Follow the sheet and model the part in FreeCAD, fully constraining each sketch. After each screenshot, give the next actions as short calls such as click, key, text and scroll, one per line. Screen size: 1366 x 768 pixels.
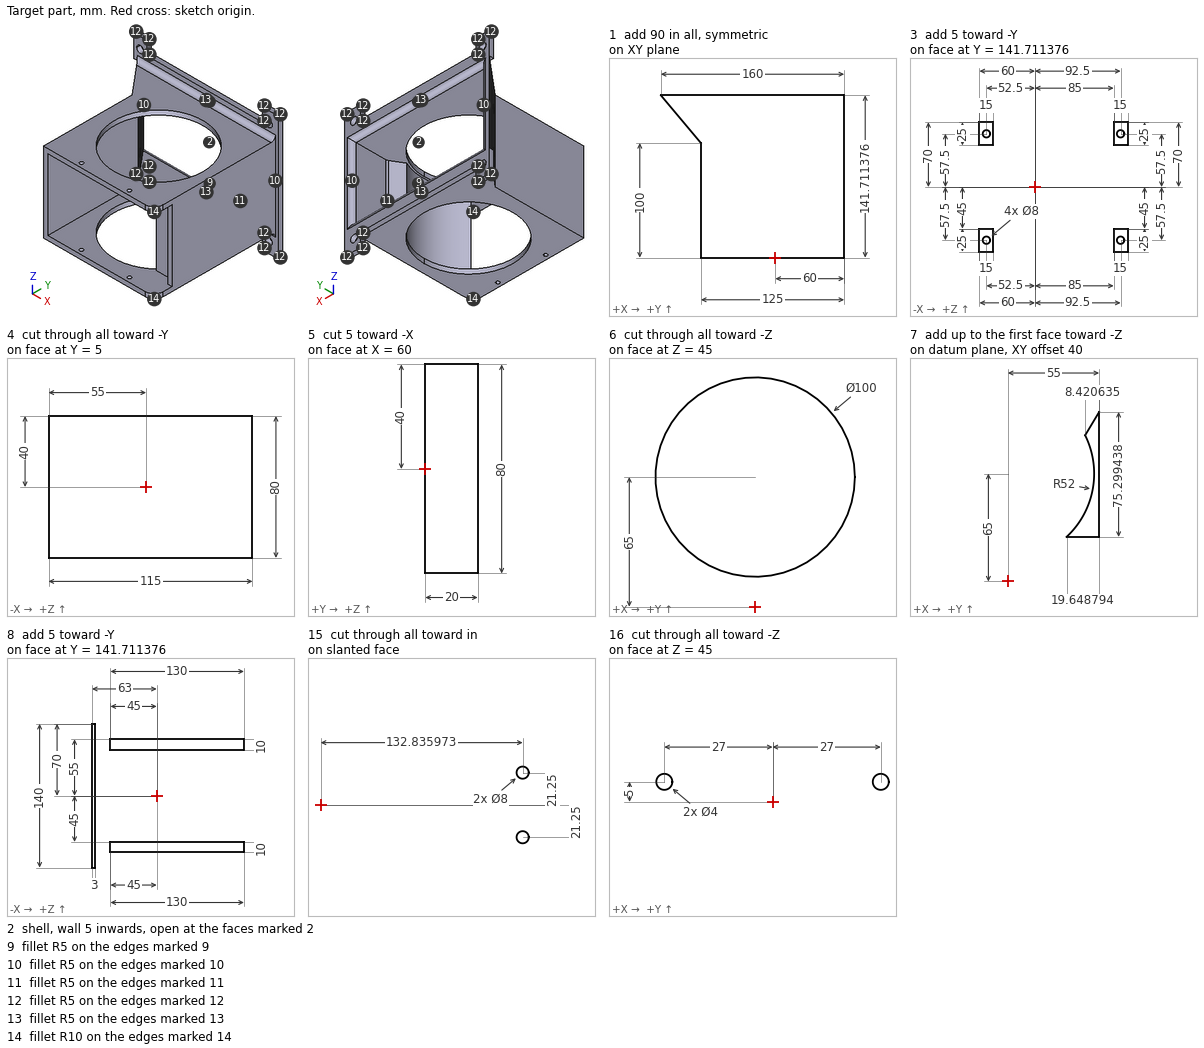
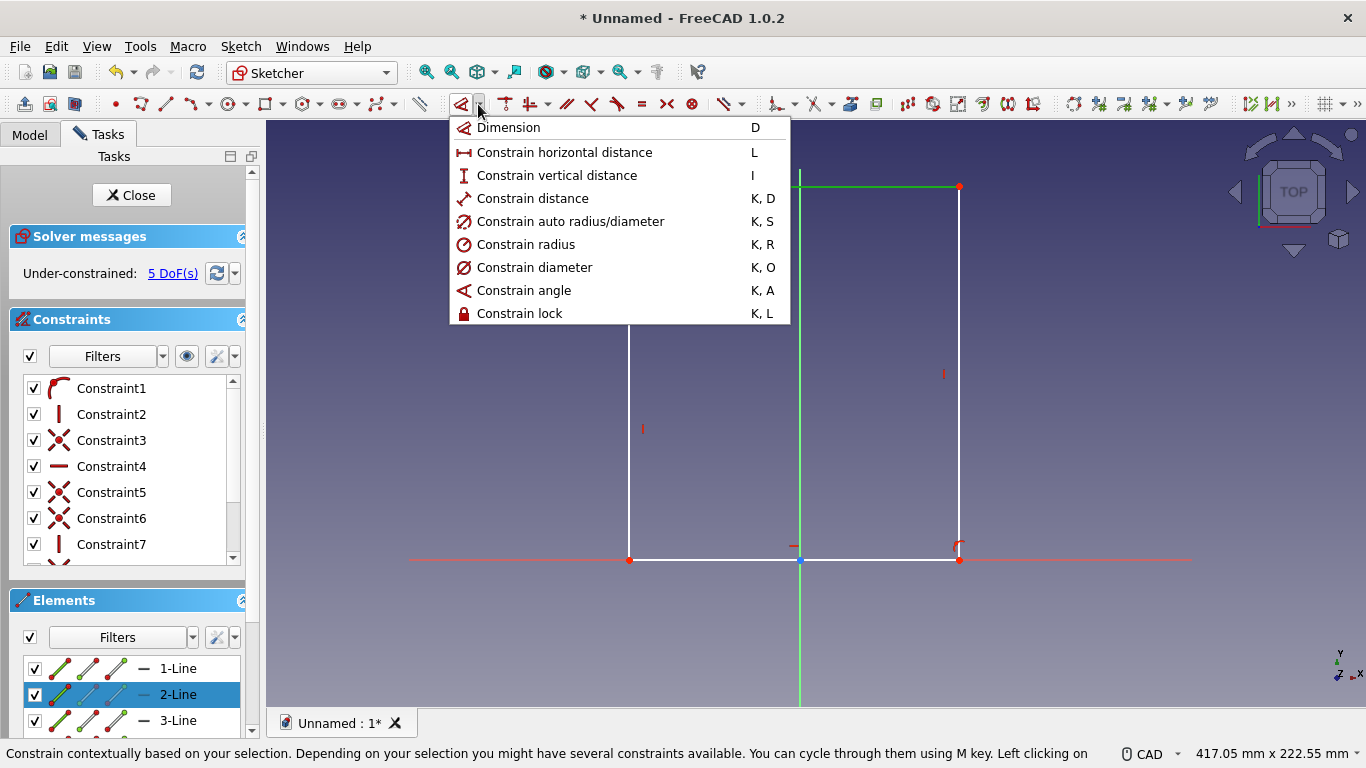
click(620, 152)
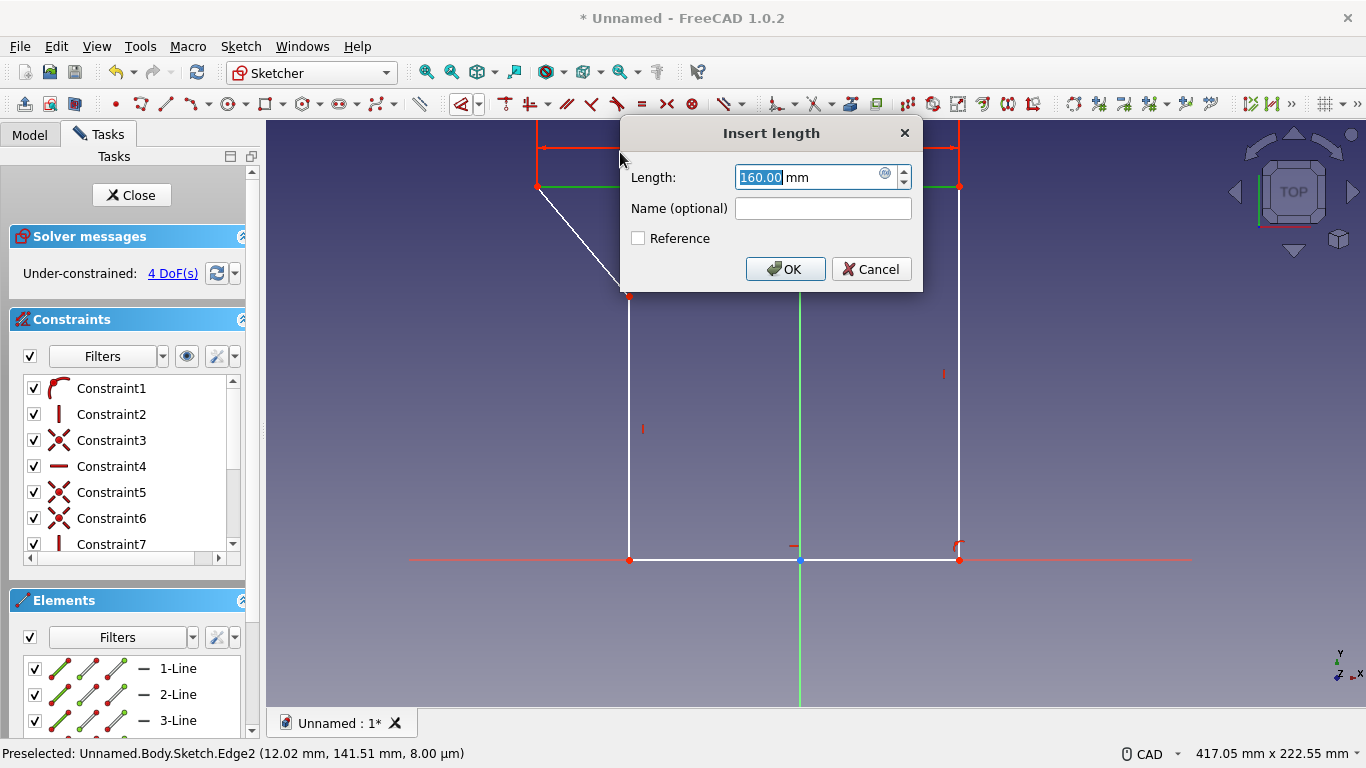
text(160)
key(Return)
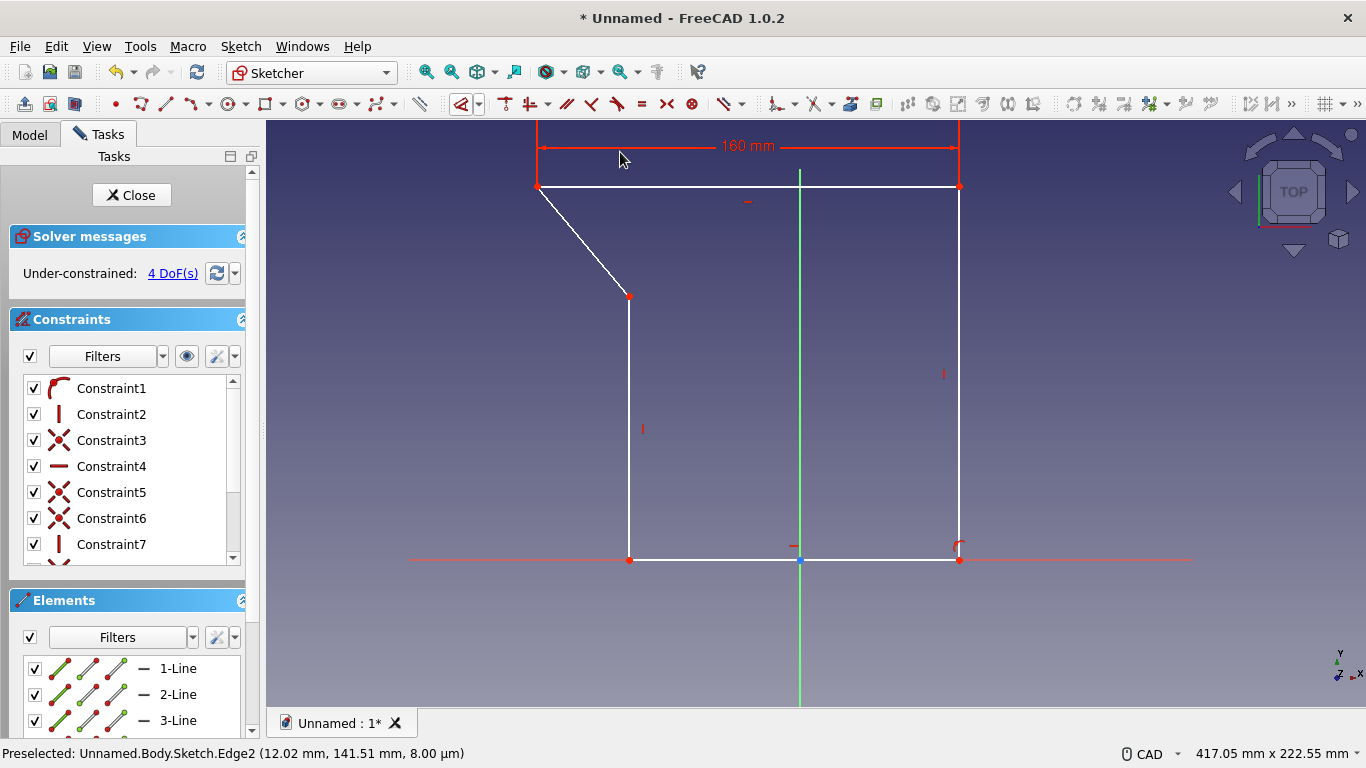
click(629, 376)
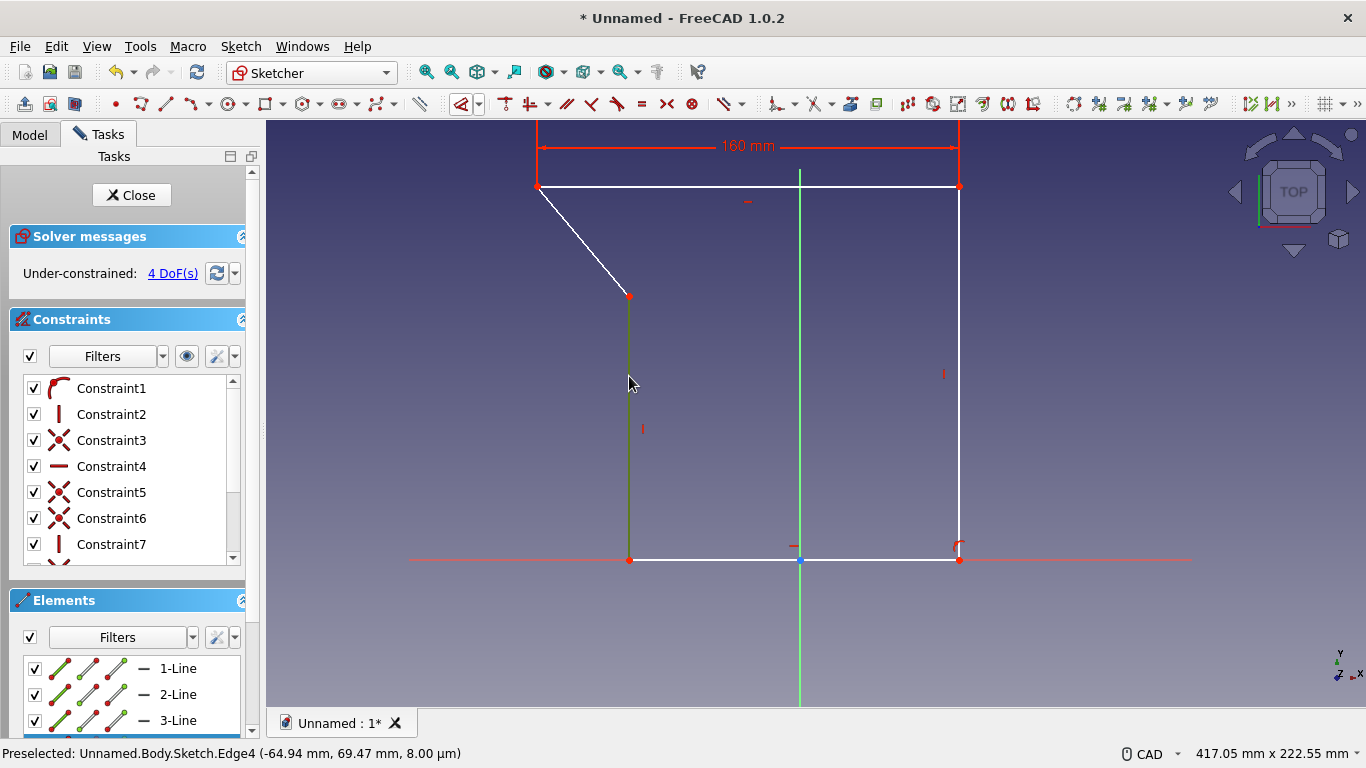
click(478, 104)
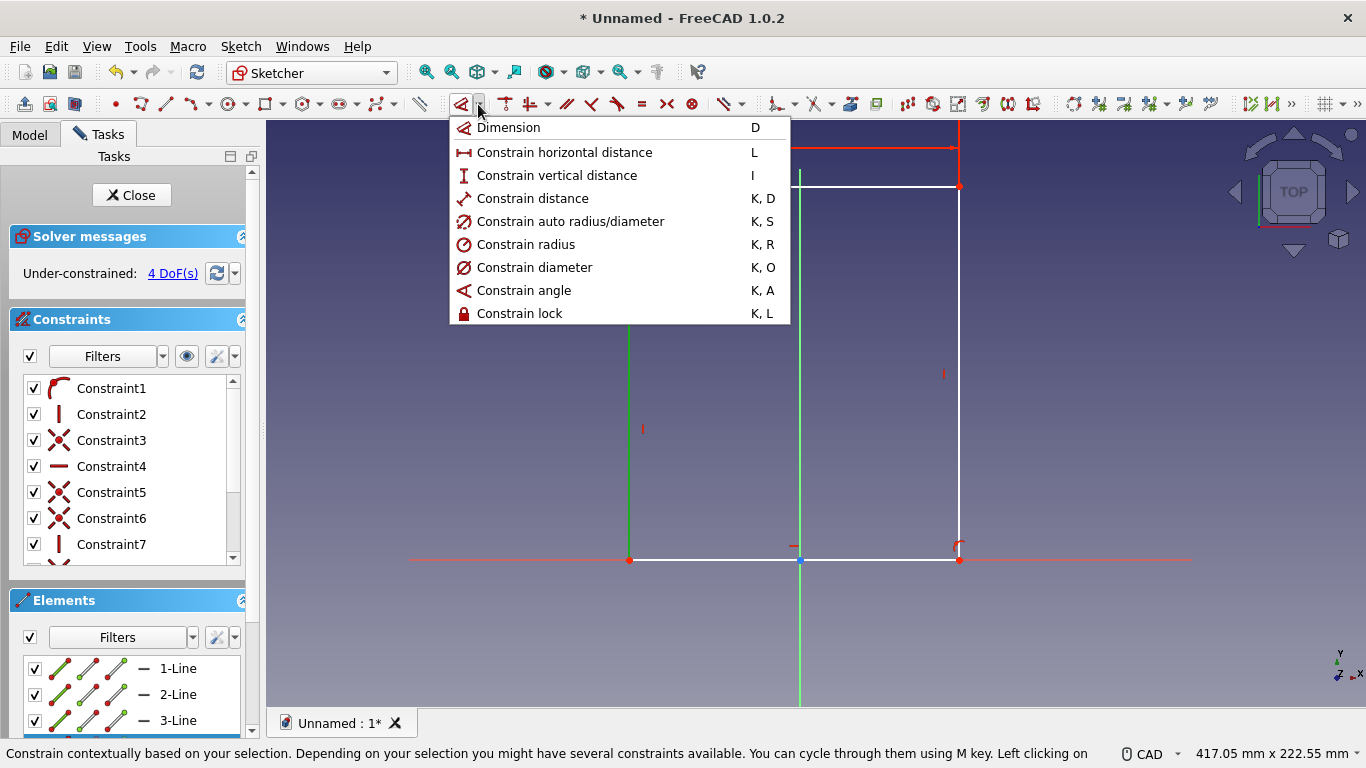
click(620, 176)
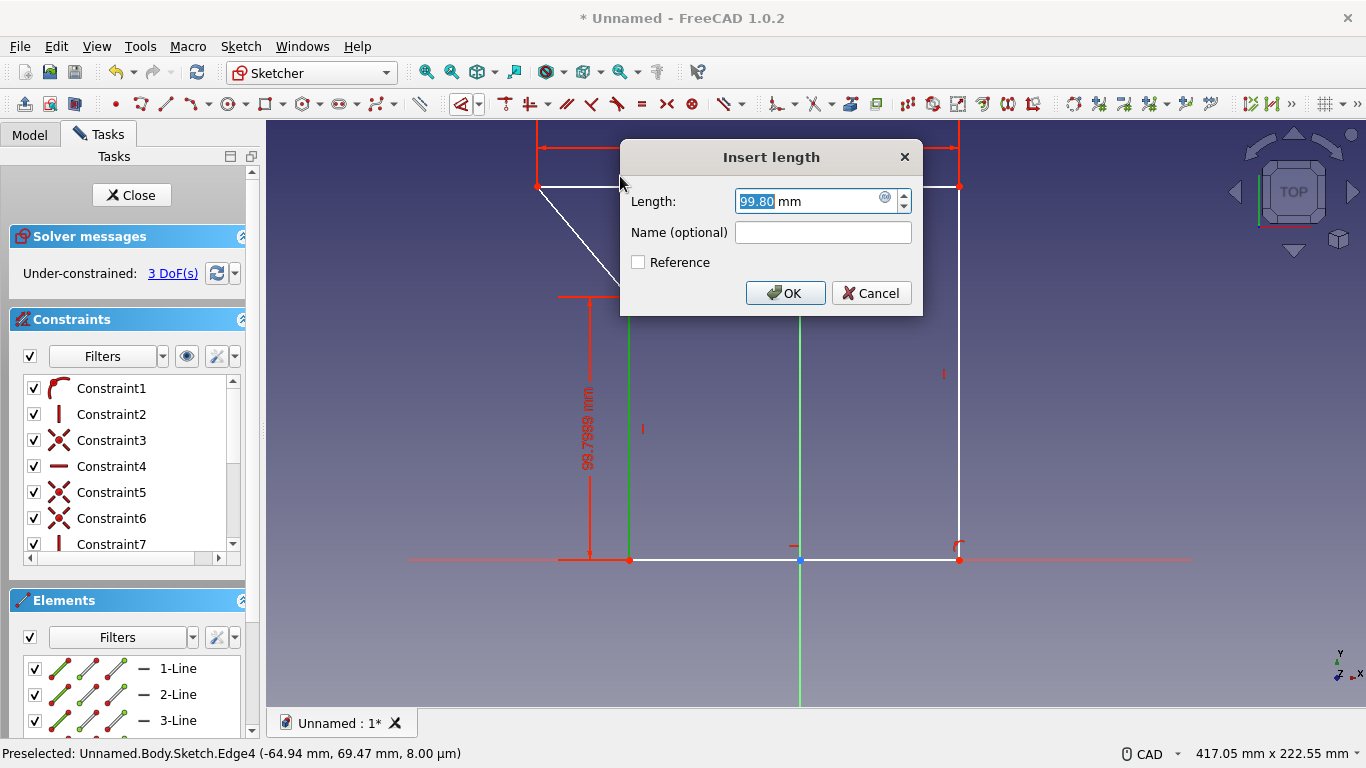
text(100)
key(Return)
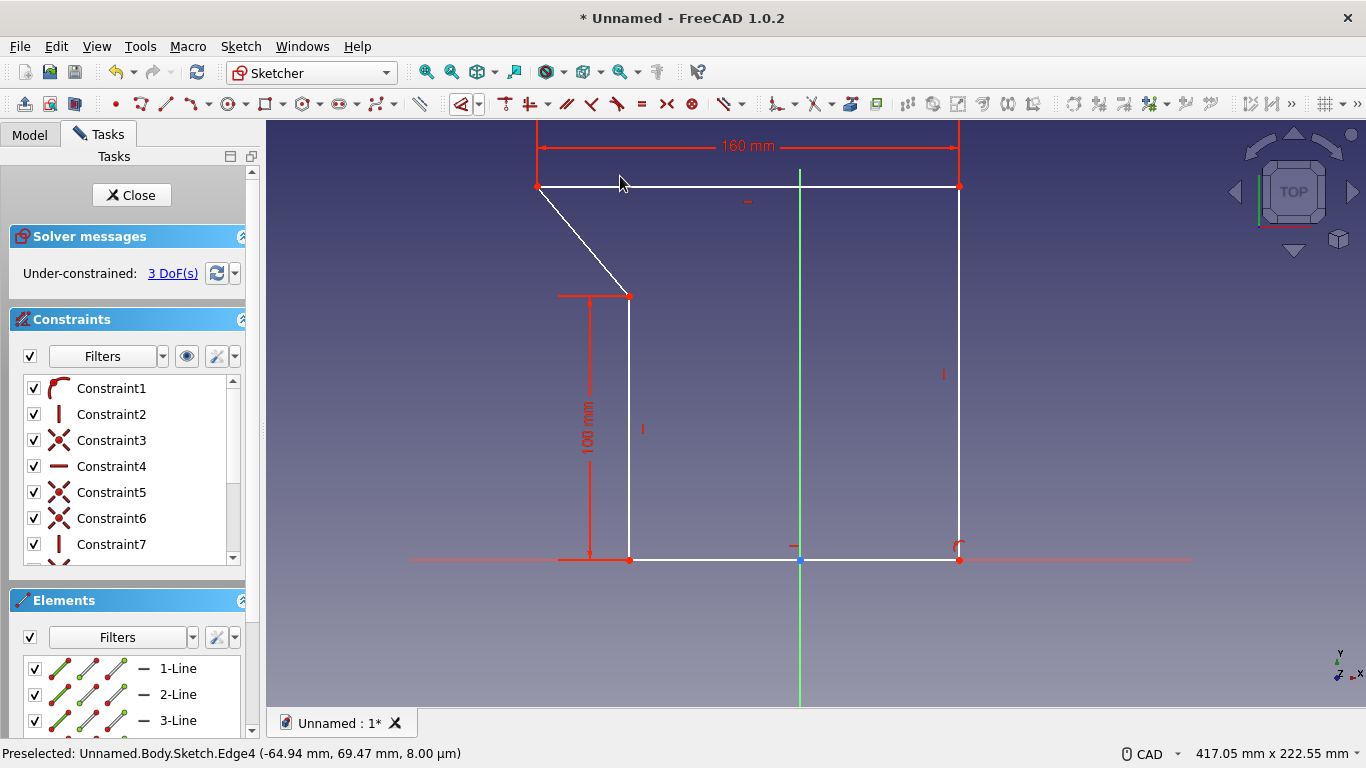
click(728, 560)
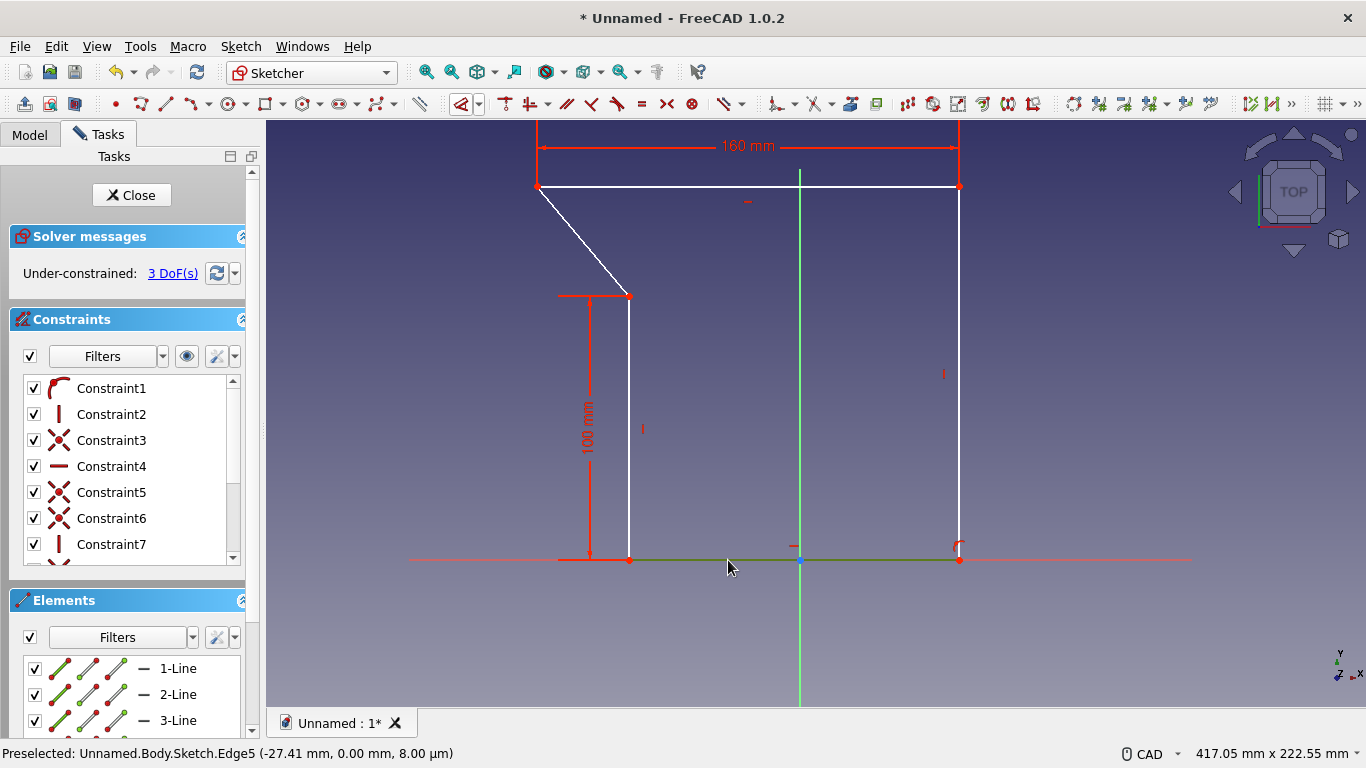
key(l)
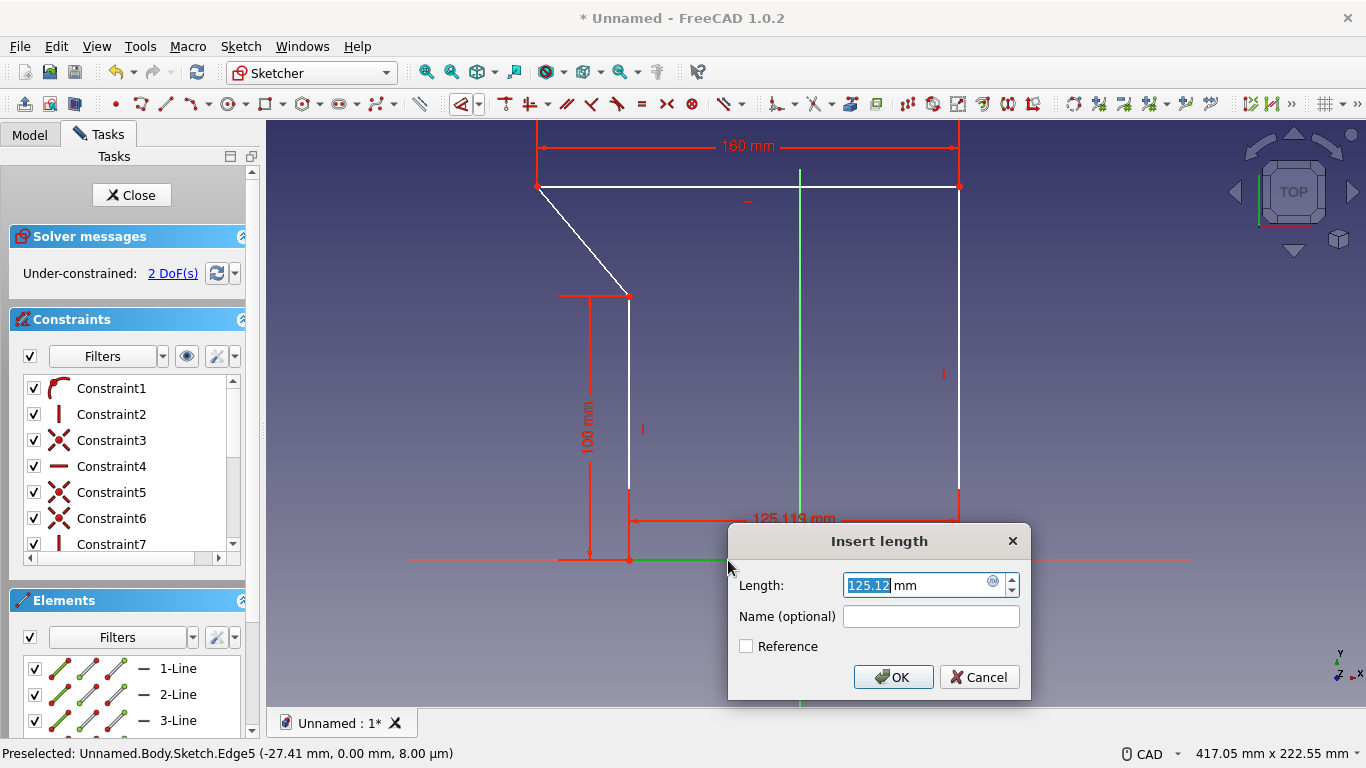
text(125)
key(Return)